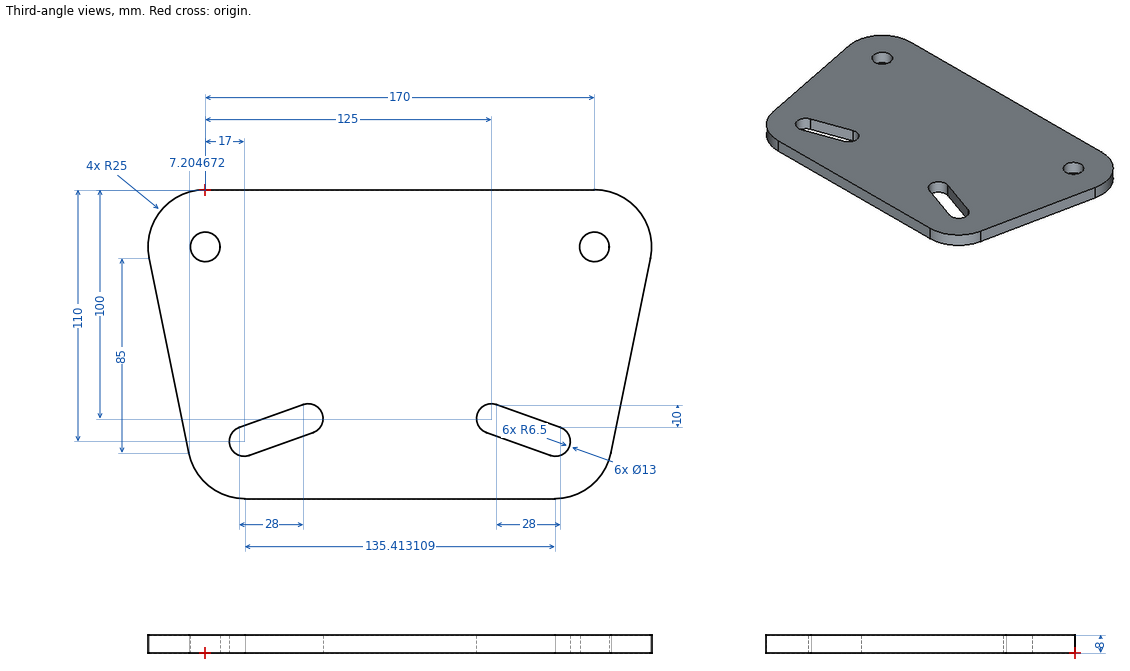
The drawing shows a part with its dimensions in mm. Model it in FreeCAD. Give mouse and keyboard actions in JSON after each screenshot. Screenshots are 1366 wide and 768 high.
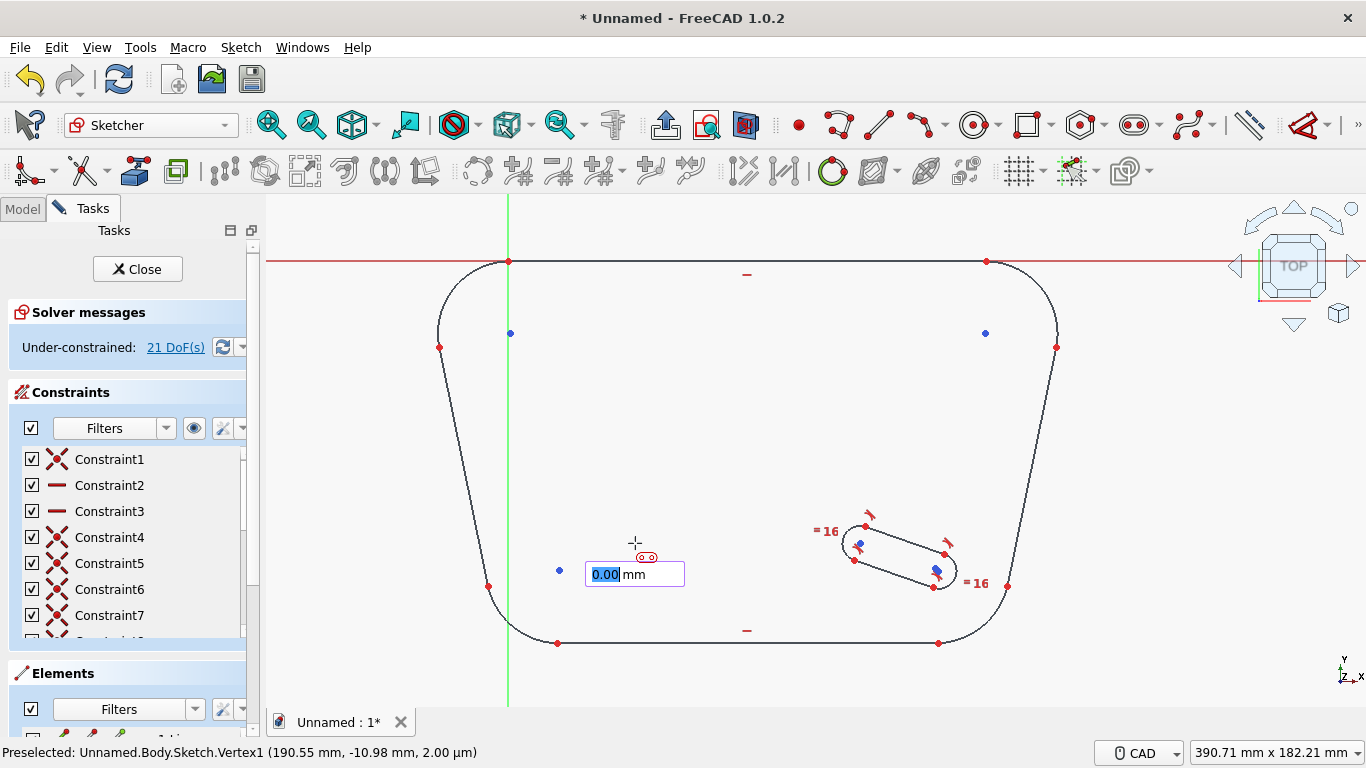
{"action": "left_click", "coordinate": [589, 540]}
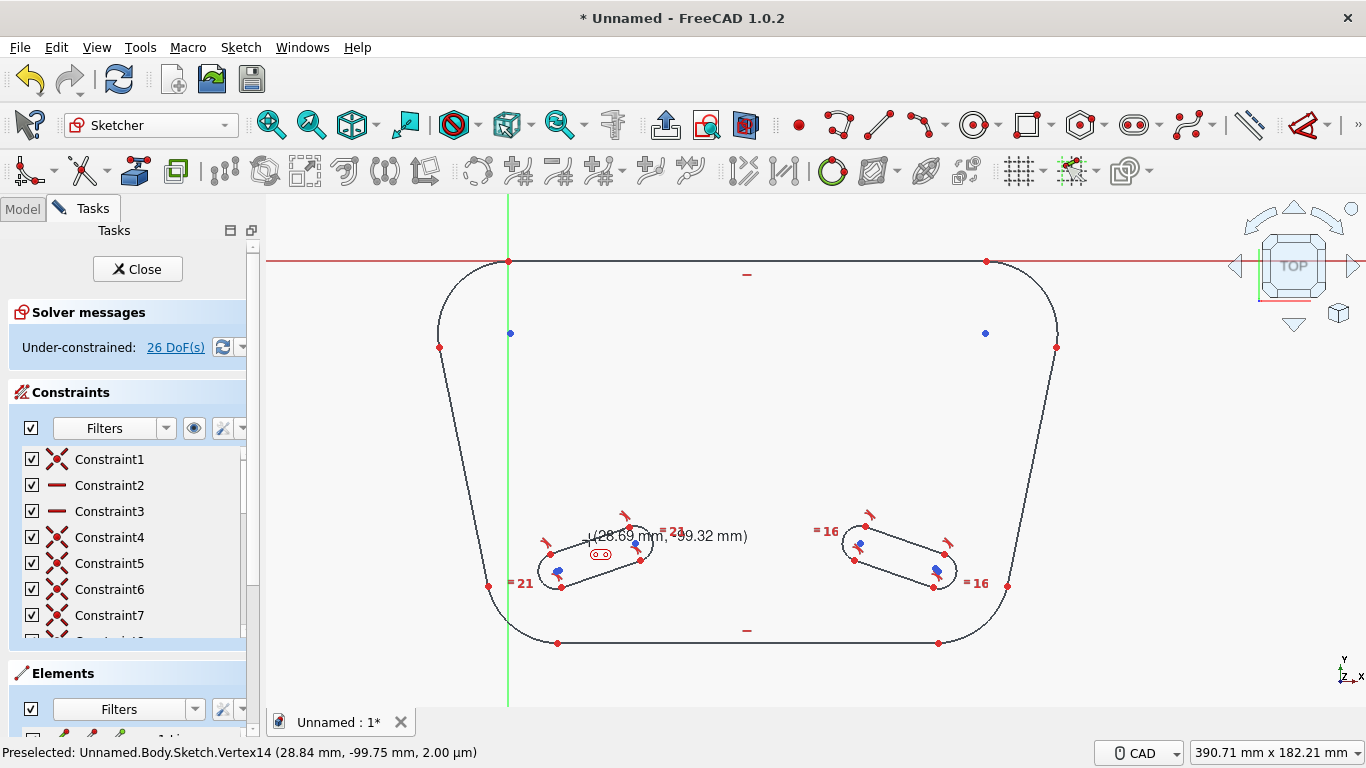
{"action": "left_click", "coordinate": [974, 126]}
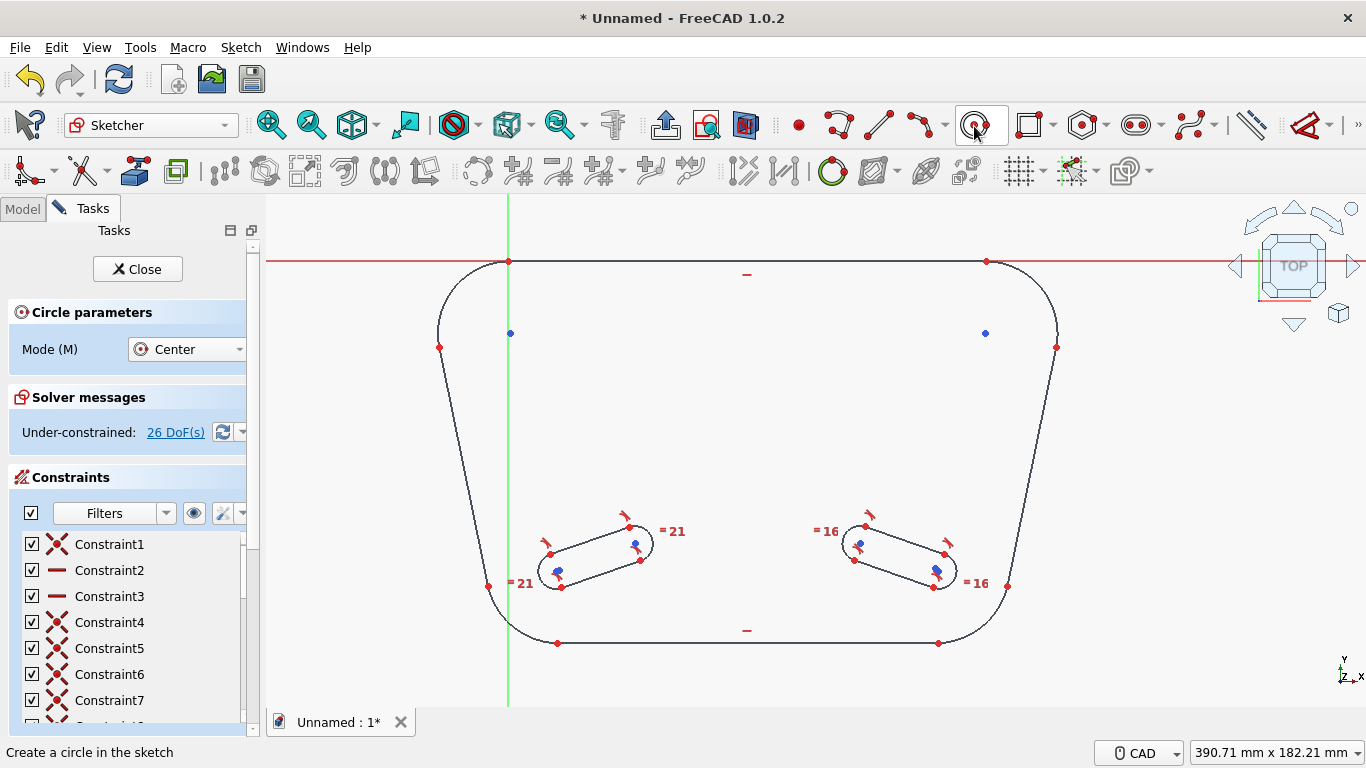
{"action": "scroll", "coordinate": [987, 332], "scroll_direction": "up", "scroll_amount": 2}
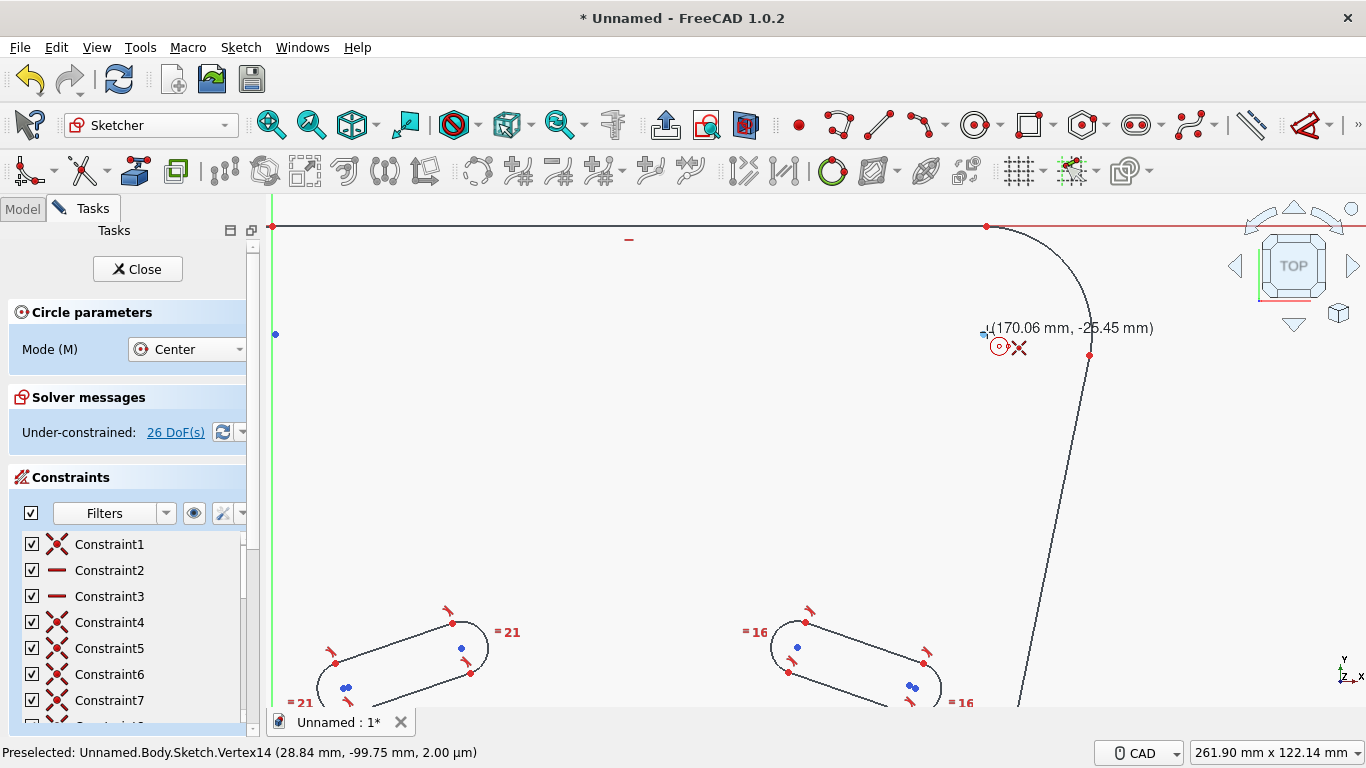
{"action": "left_click", "coordinate": [986, 331]}
{"action": "left_click", "coordinate": [1006, 312]}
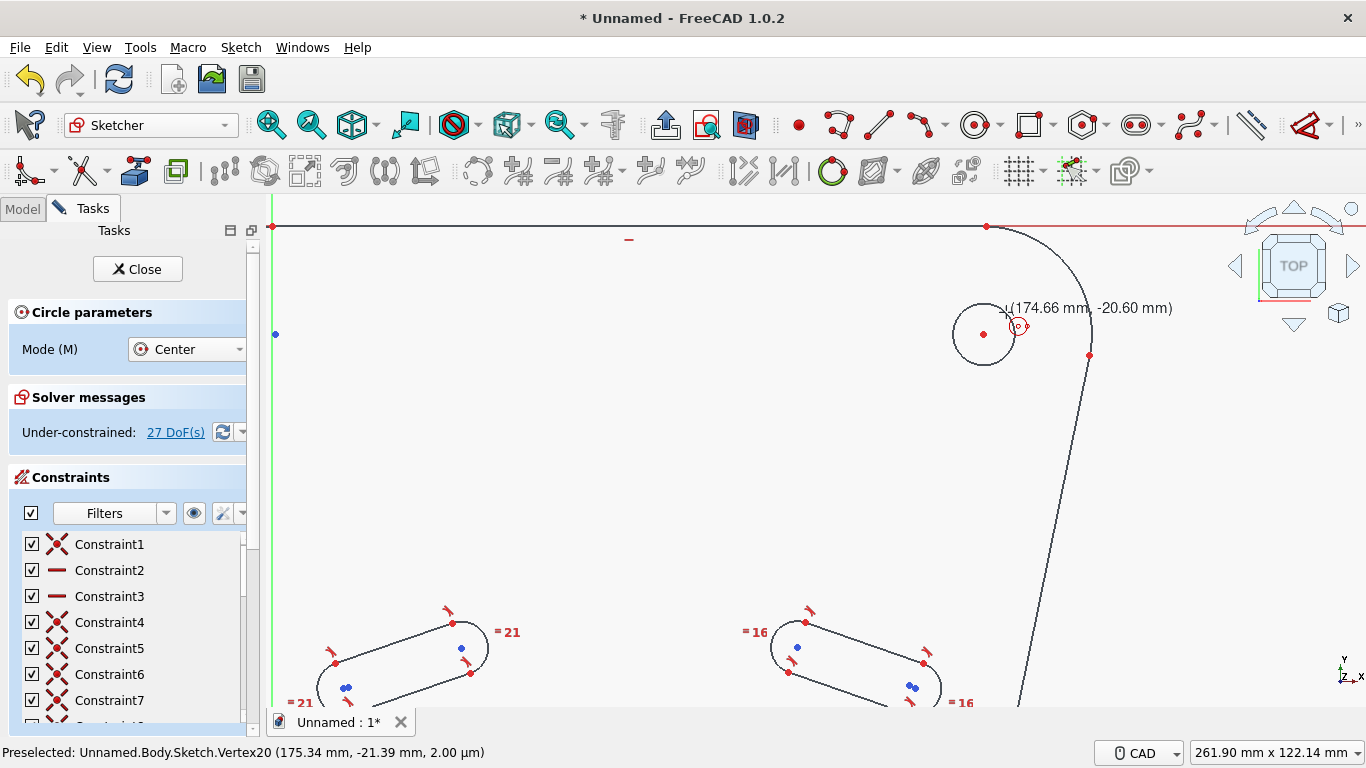
{"action": "scroll", "coordinate": [891, 378], "scroll_direction": "down", "scroll_amount": 3}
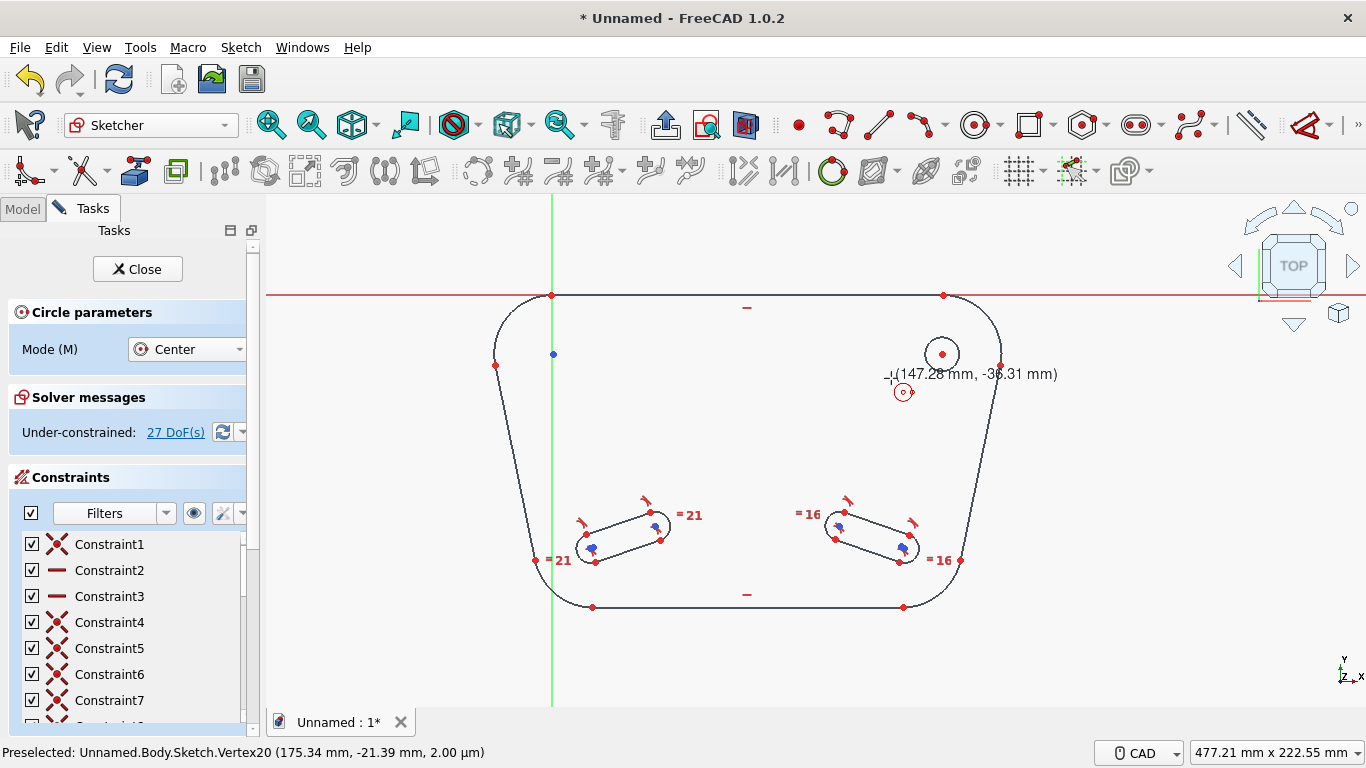
{"action": "scroll", "coordinate": [552, 353], "scroll_direction": "up", "scroll_amount": 3}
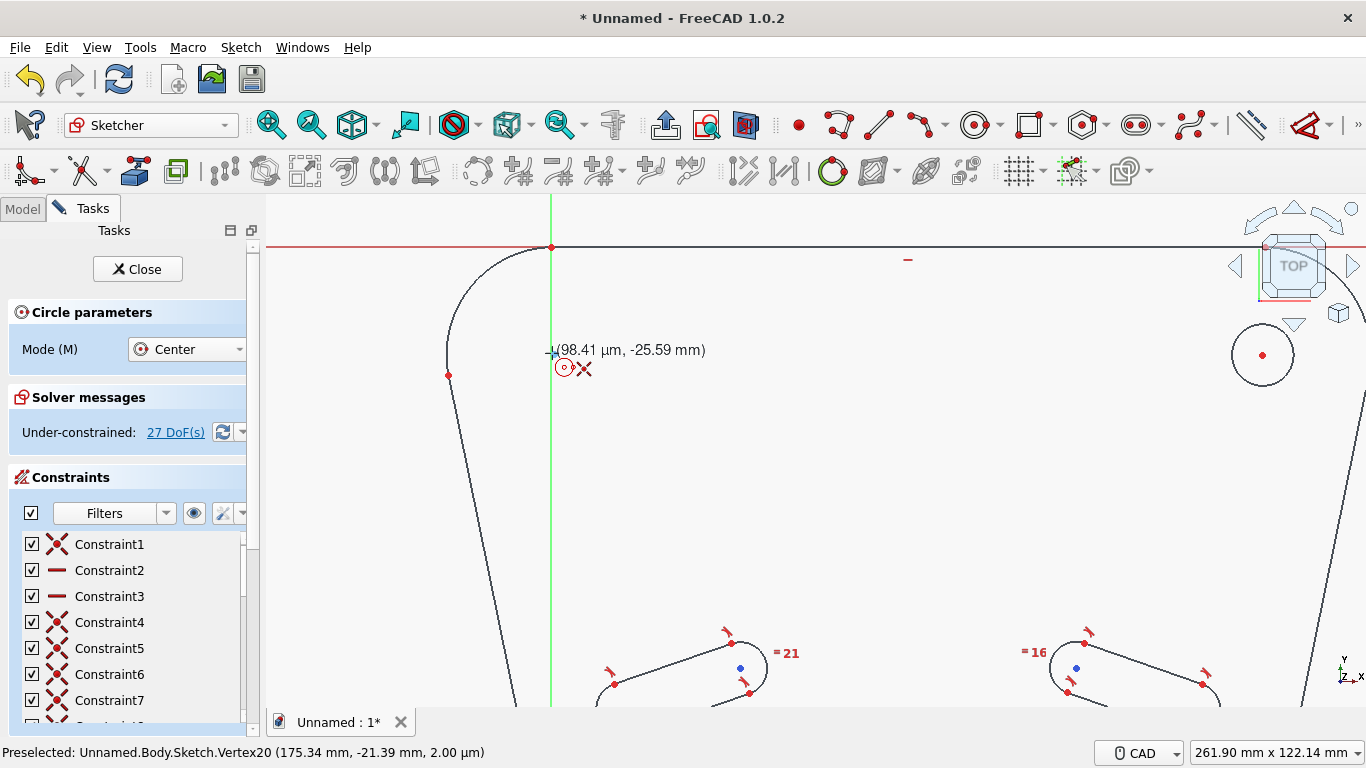
{"action": "left_click", "coordinate": [551, 352]}
{"action": "left_click", "coordinate": [571, 333]}
{"action": "key", "text": "Escape"}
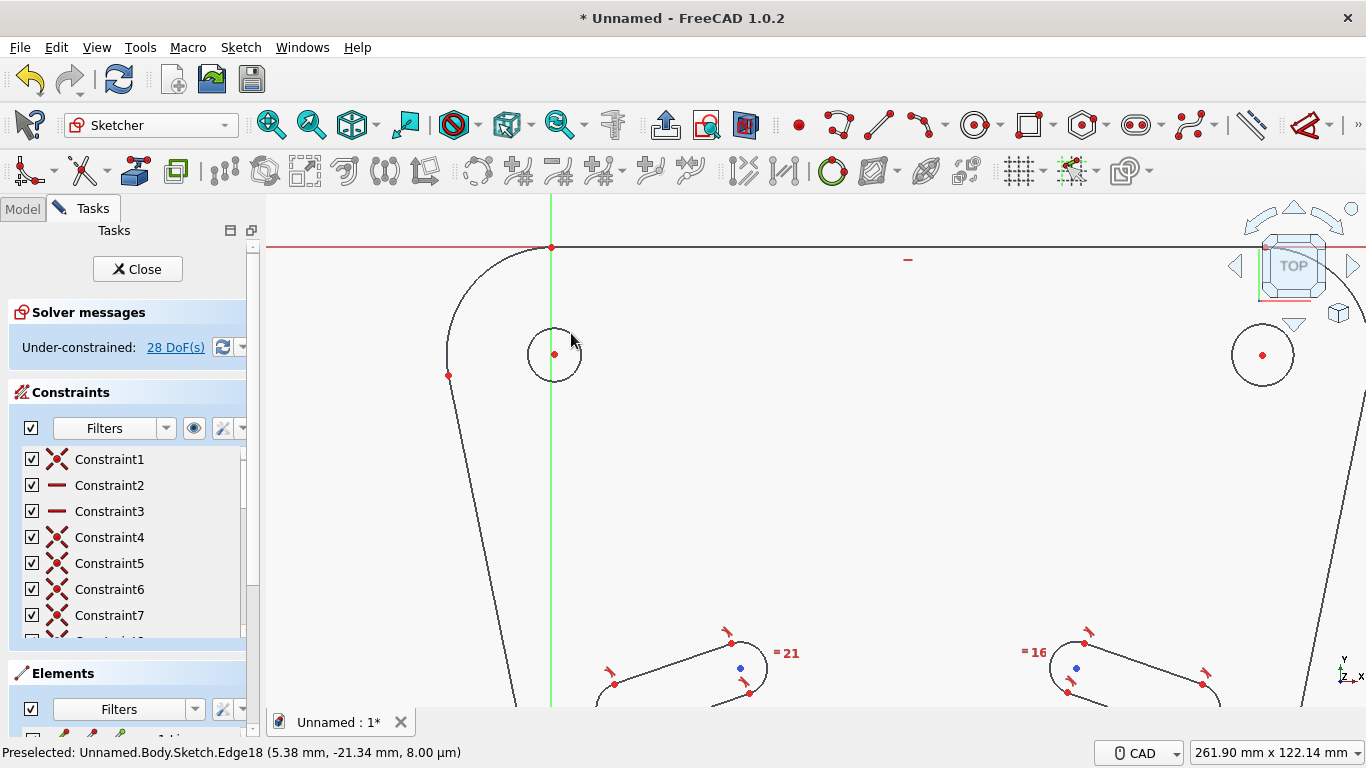
{"action": "left_click", "coordinate": [1051, 247]}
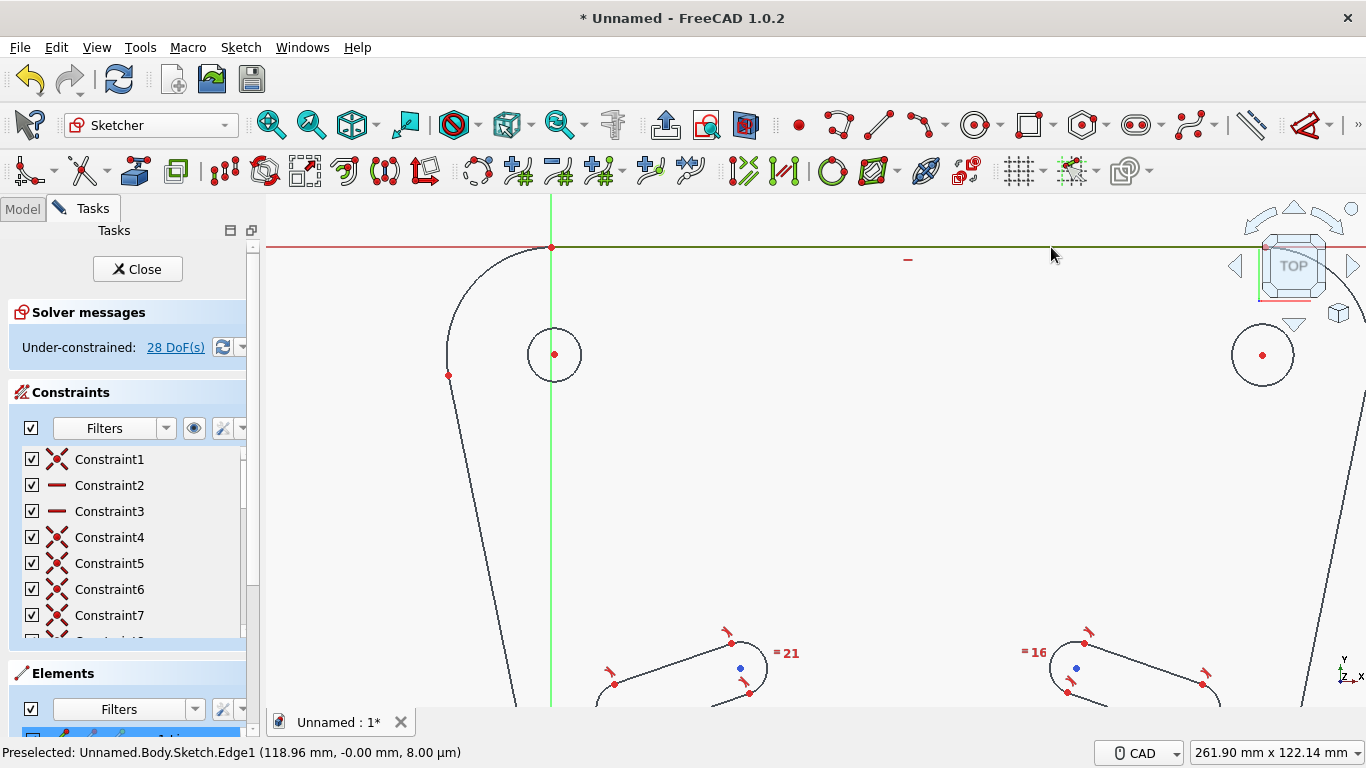
{"action": "left_click", "coordinate": [498, 263]}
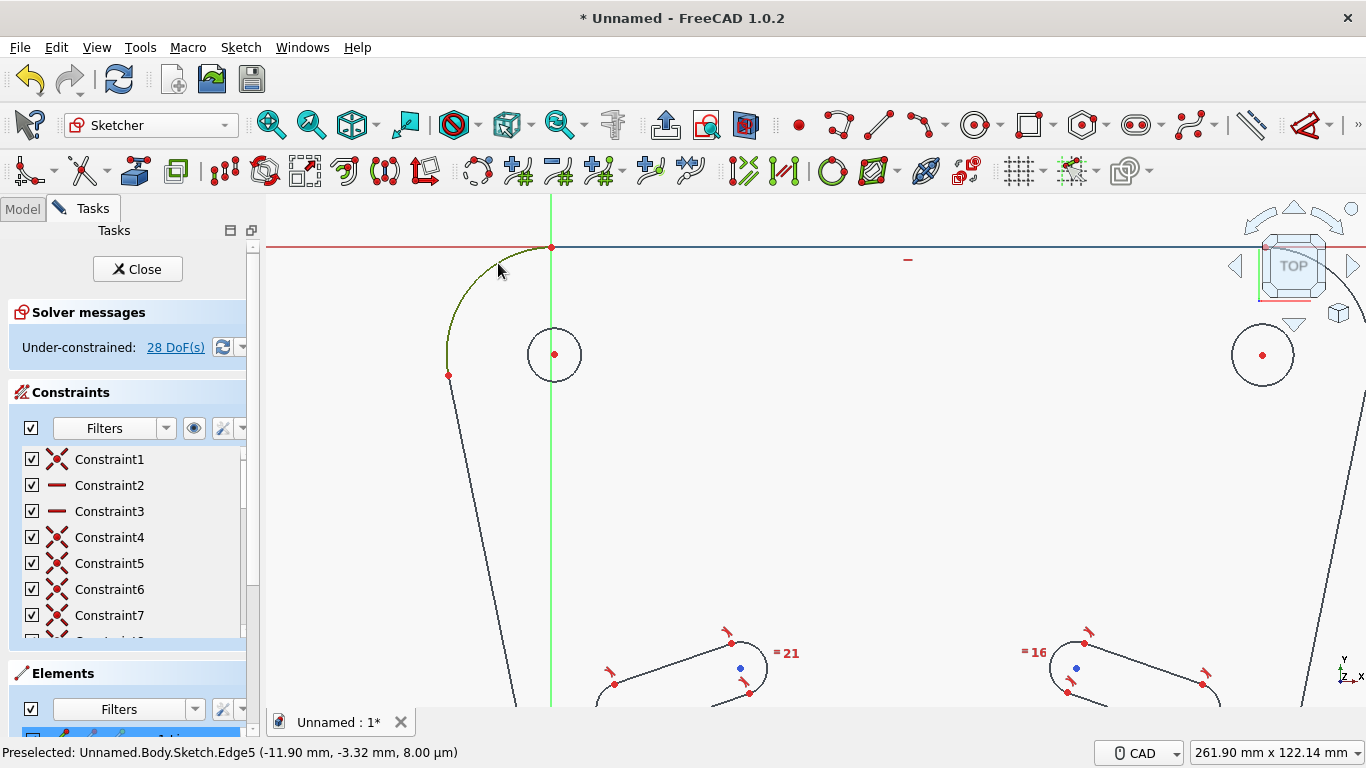
{"action": "key", "text": "t"}